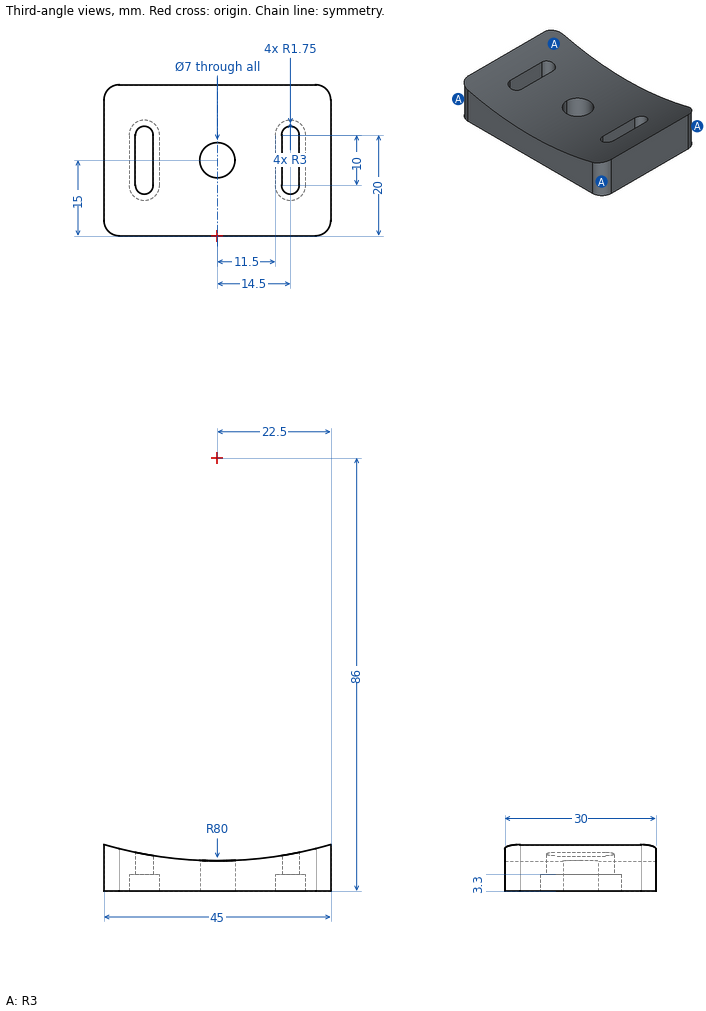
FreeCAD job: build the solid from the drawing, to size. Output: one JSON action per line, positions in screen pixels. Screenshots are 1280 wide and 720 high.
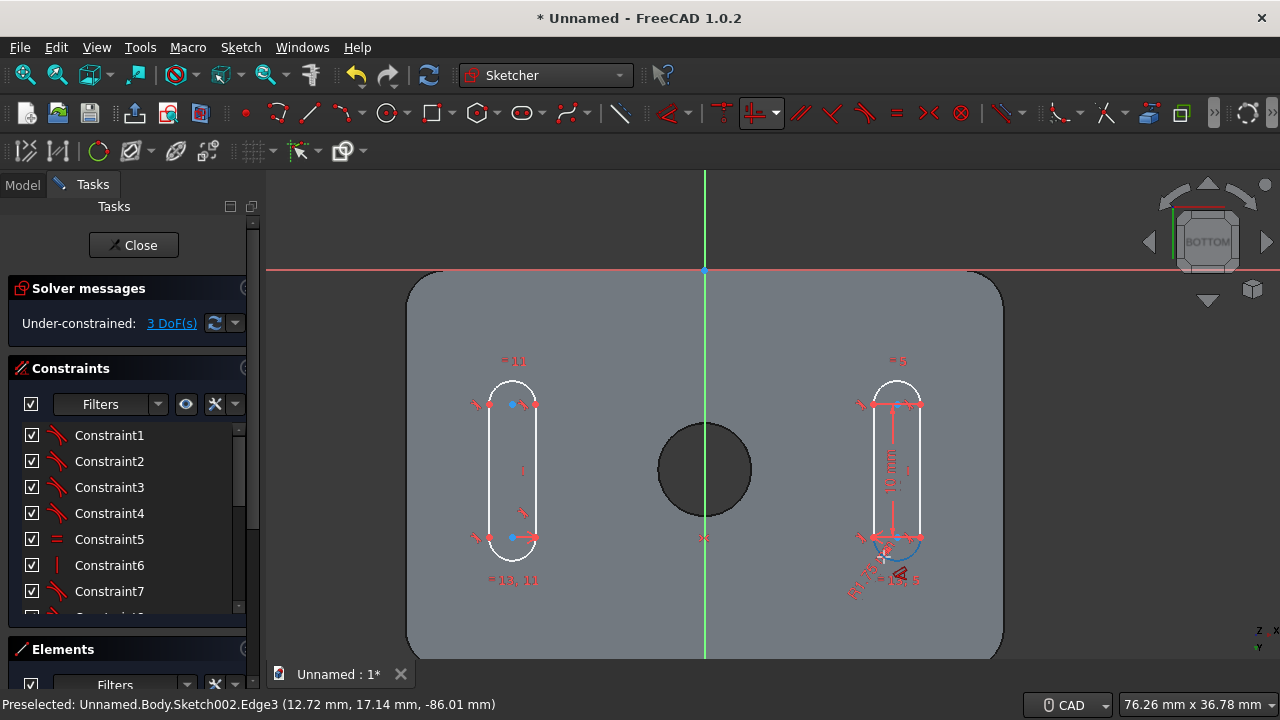
{"action": "left_click", "coordinate": [489, 498]}
{"action": "left_click", "coordinate": [455, 471]}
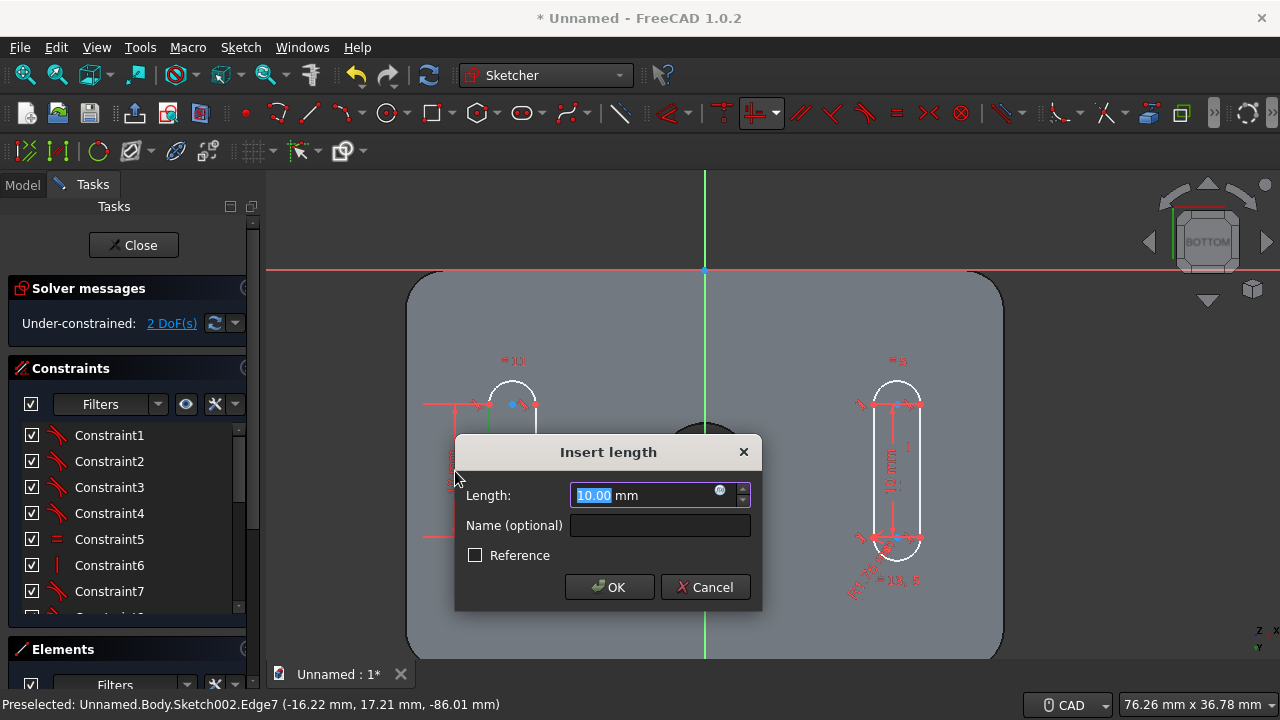
{"action": "type", "text": "10"}
{"action": "key", "text": "Return"}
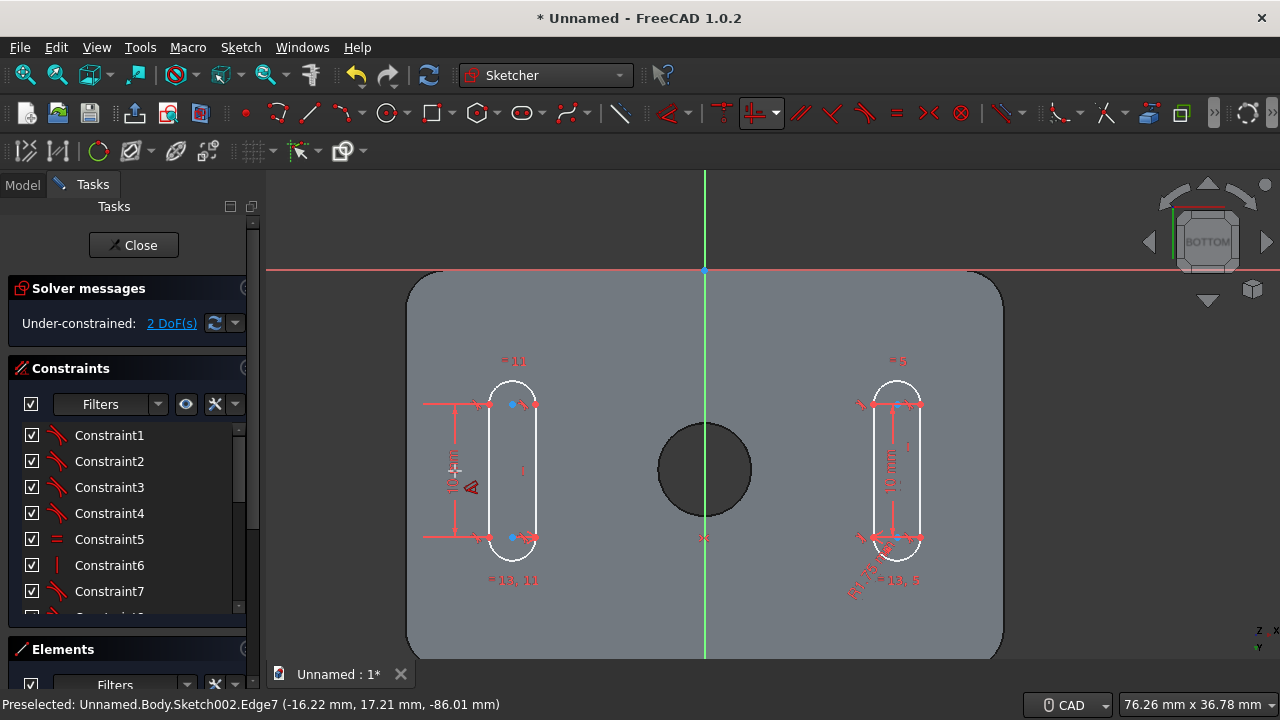
{"action": "left_click", "coordinate": [874, 537]}
{"action": "left_click", "coordinate": [908, 342]}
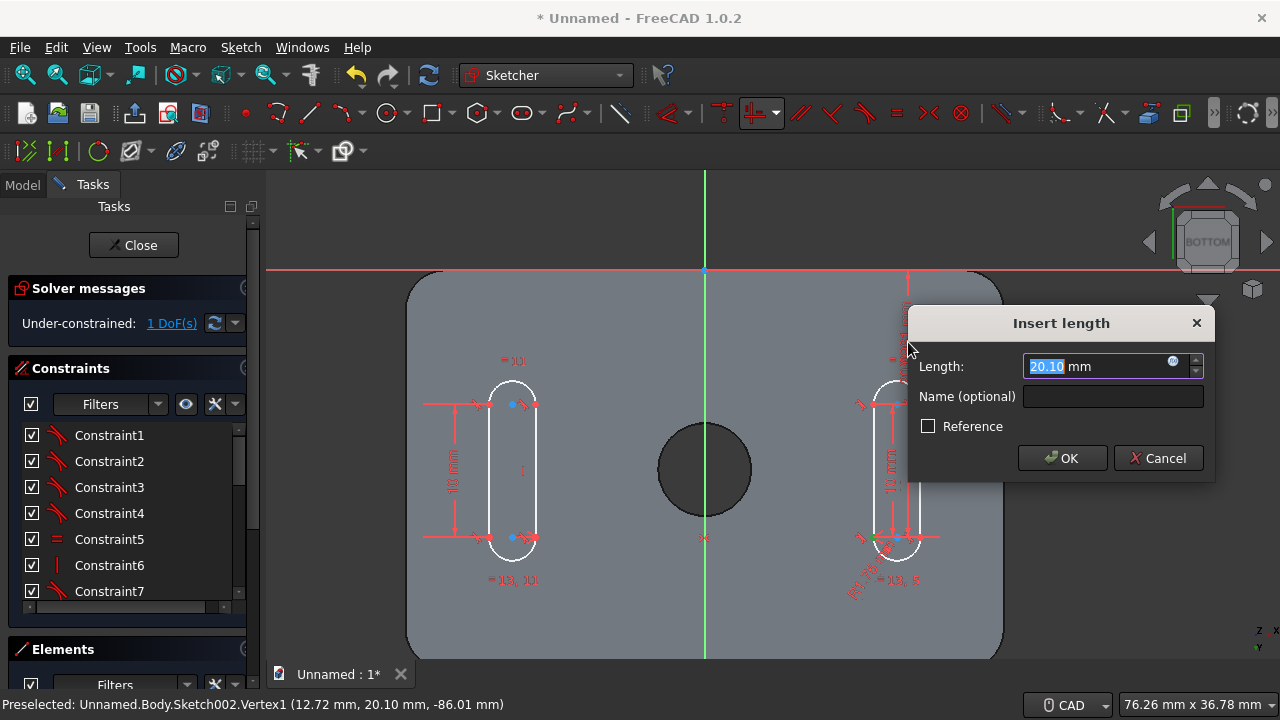
{"action": "type", "text": "20"}
{"action": "key", "text": "Return"}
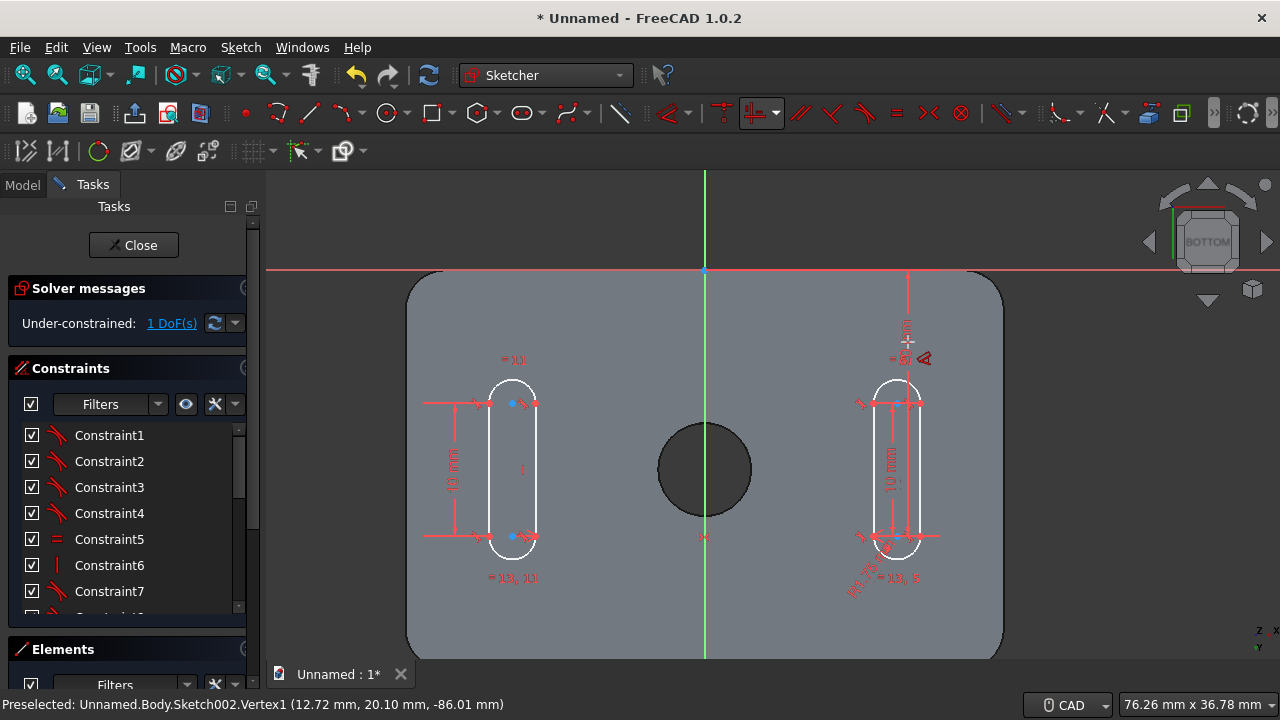
{"action": "left_click", "coordinate": [897, 536]}
{"action": "left_click", "coordinate": [801, 236]}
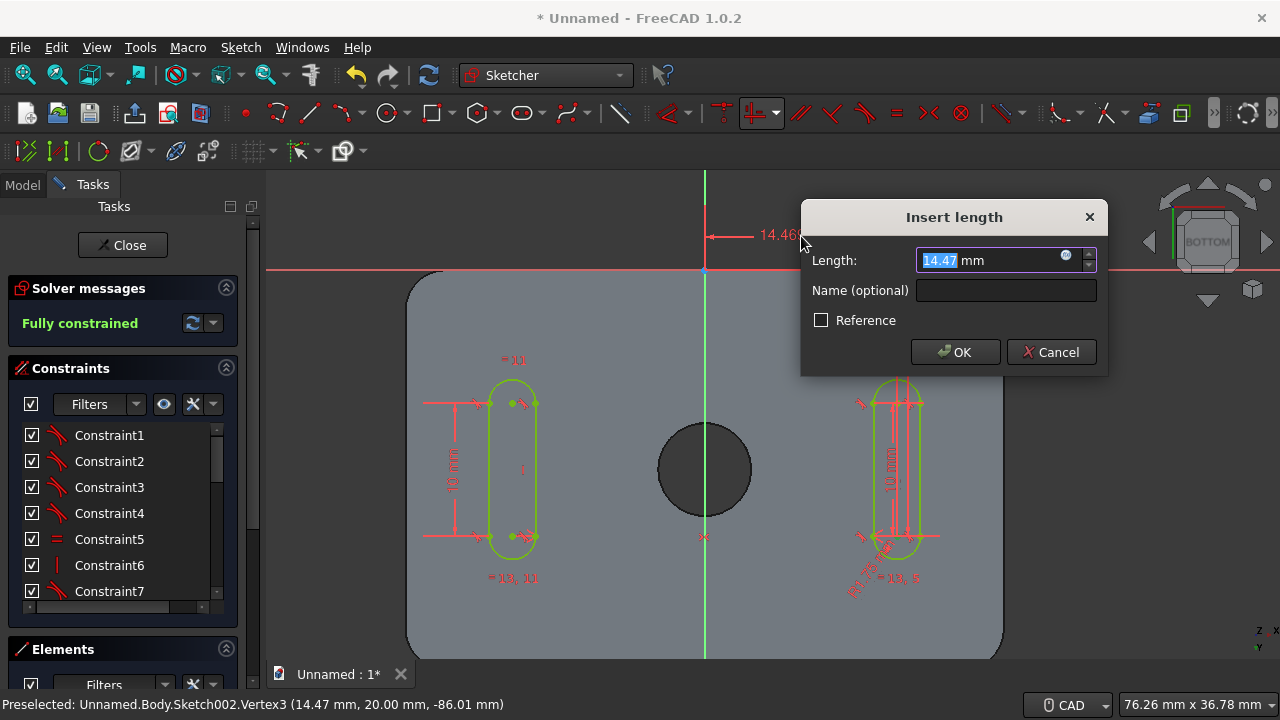
{"action": "type", "text": "14.5"}
{"action": "key", "text": "Return"}
{"action": "key", "text": "Escape"}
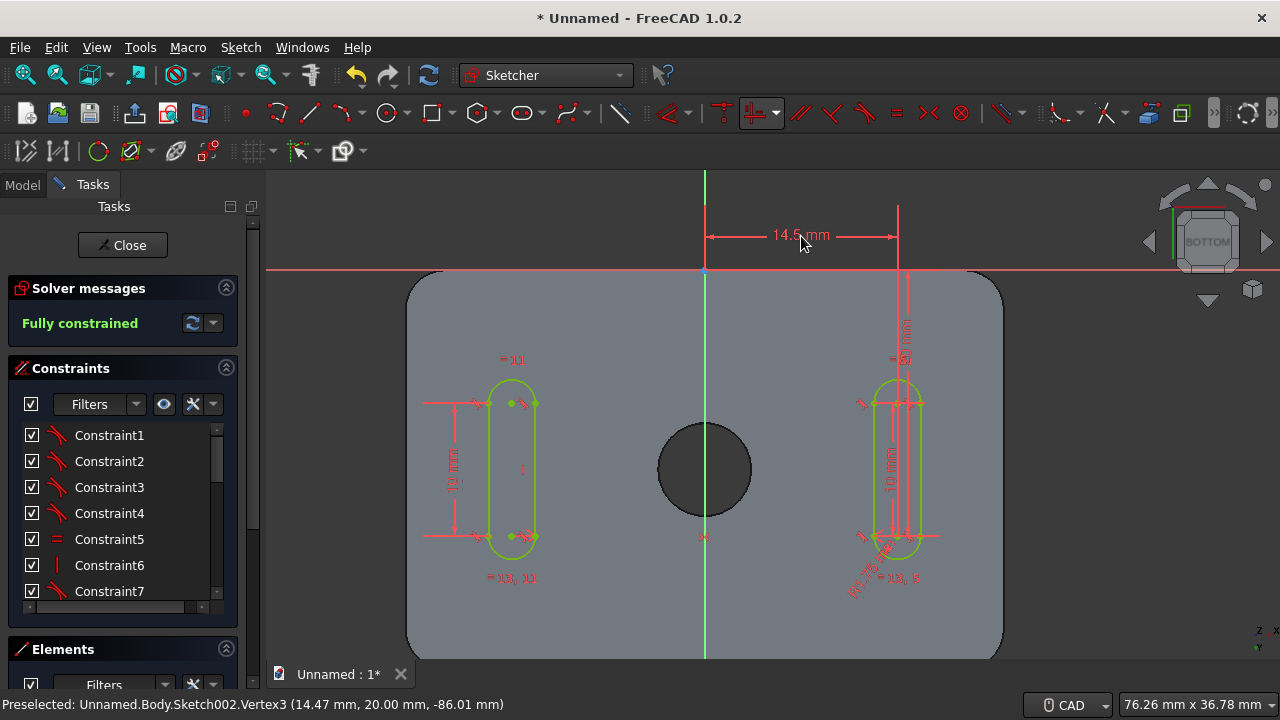
{"action": "left_click", "coordinate": [123, 245]}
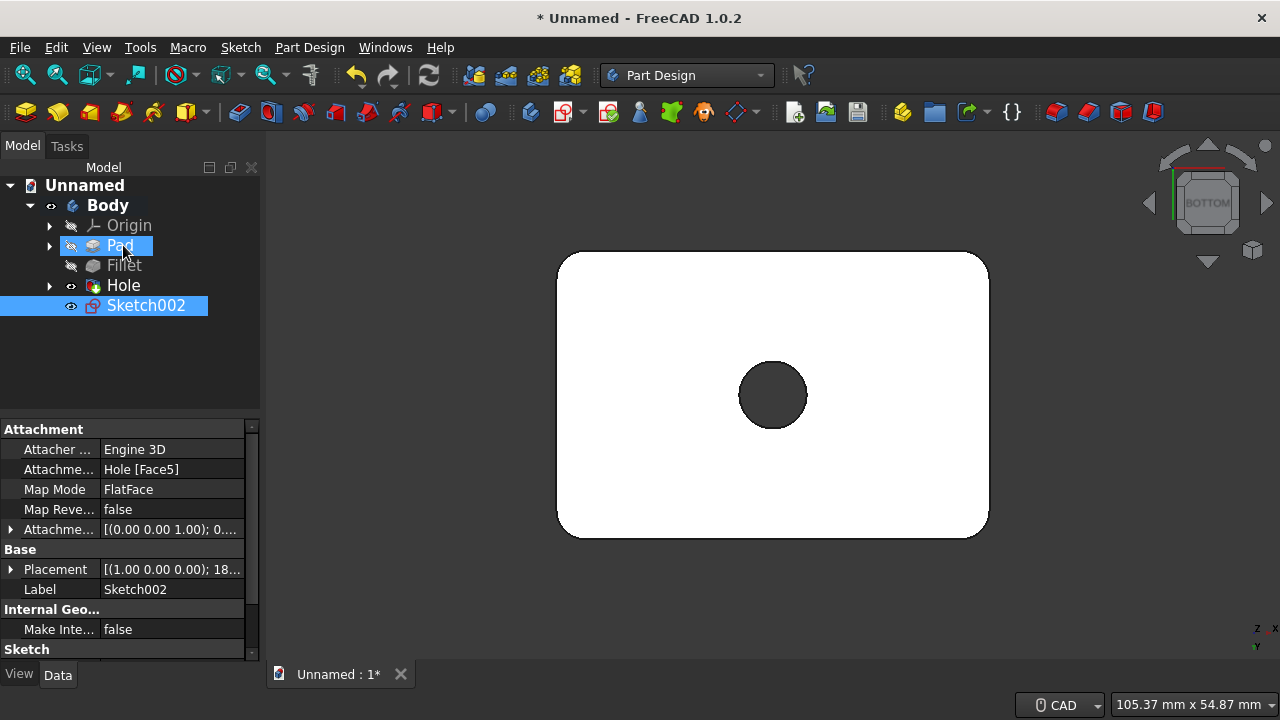
{"action": "left_click", "coordinate": [240, 112]}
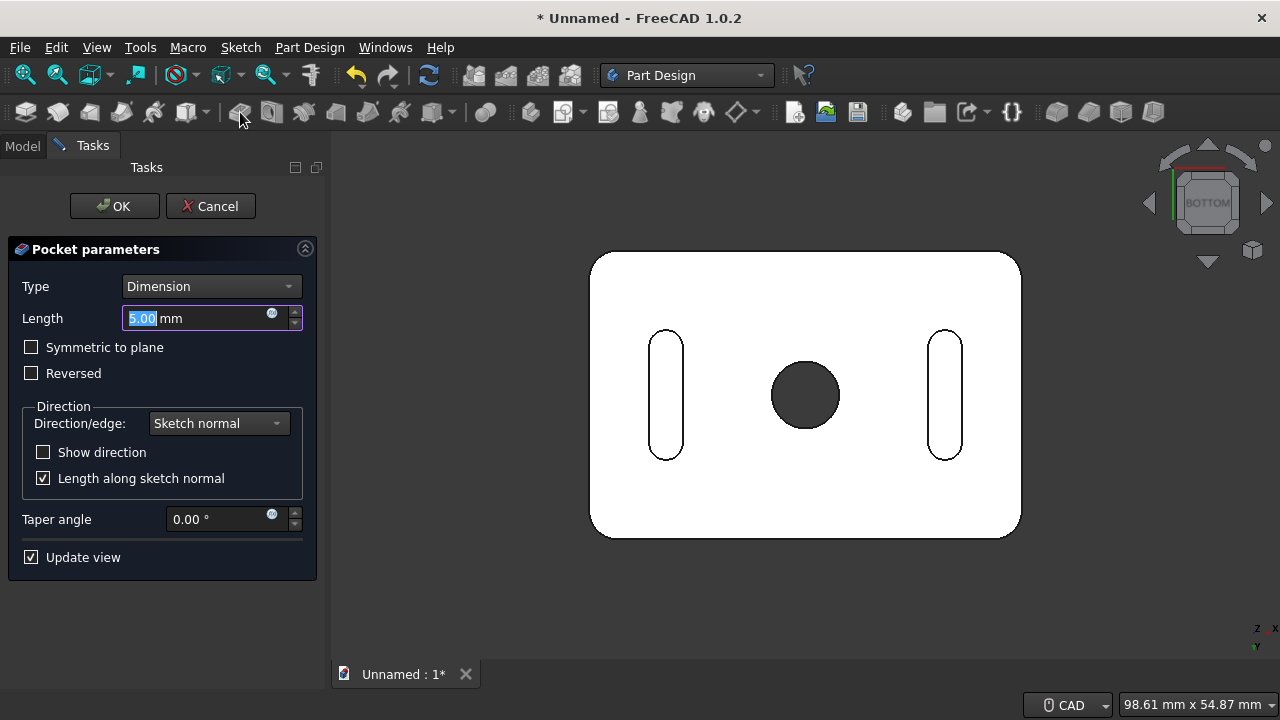
{"action": "left_click", "coordinate": [212, 286]}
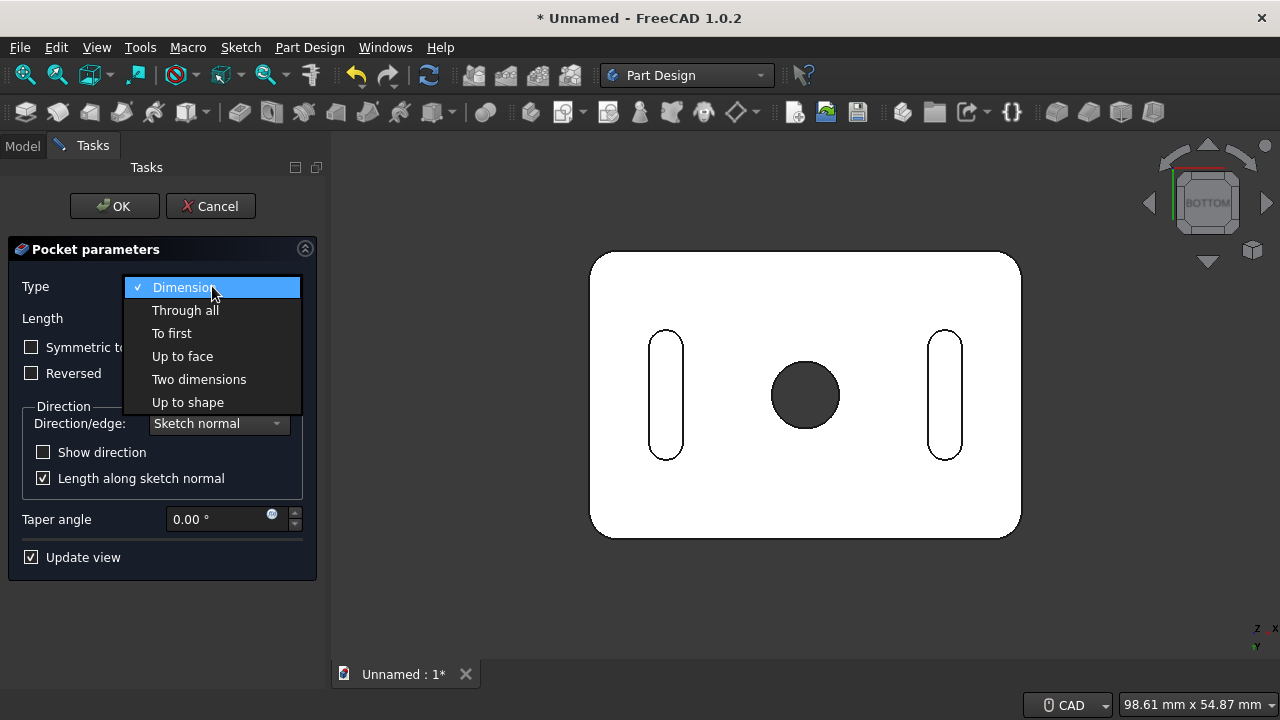
{"action": "left_click", "coordinate": [212, 310]}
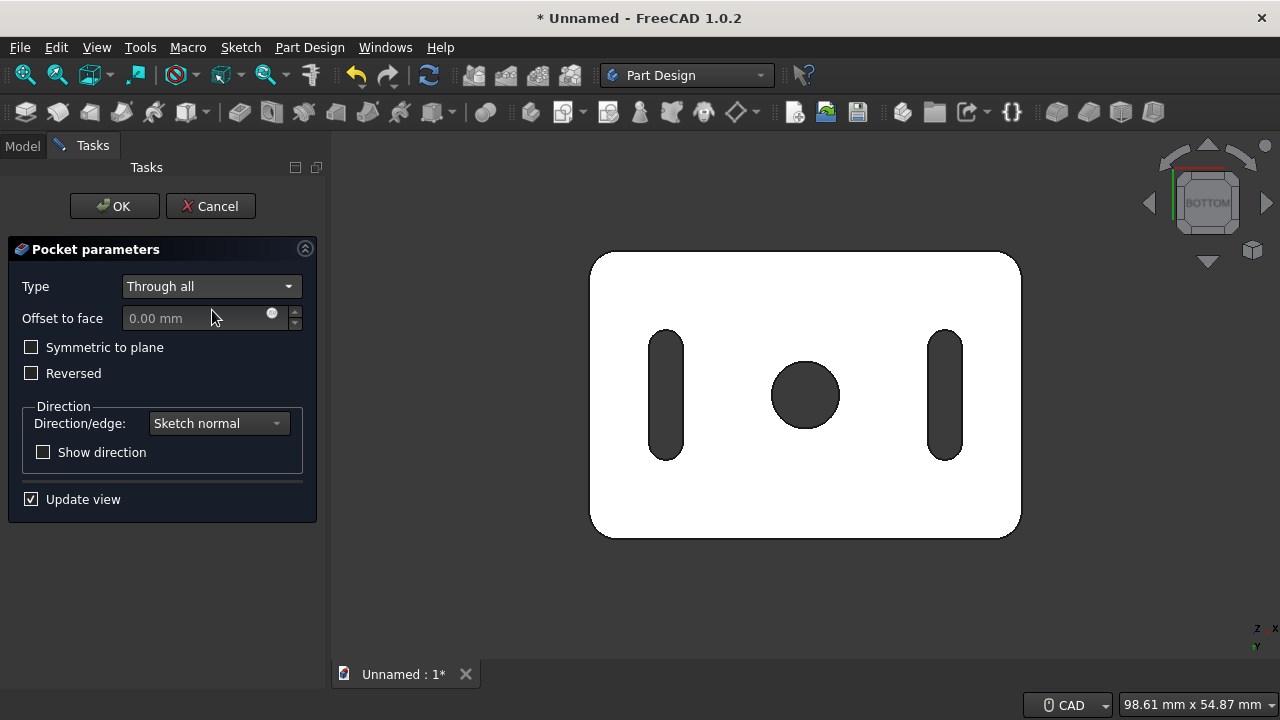
{"action": "left_click", "coordinate": [115, 206]}